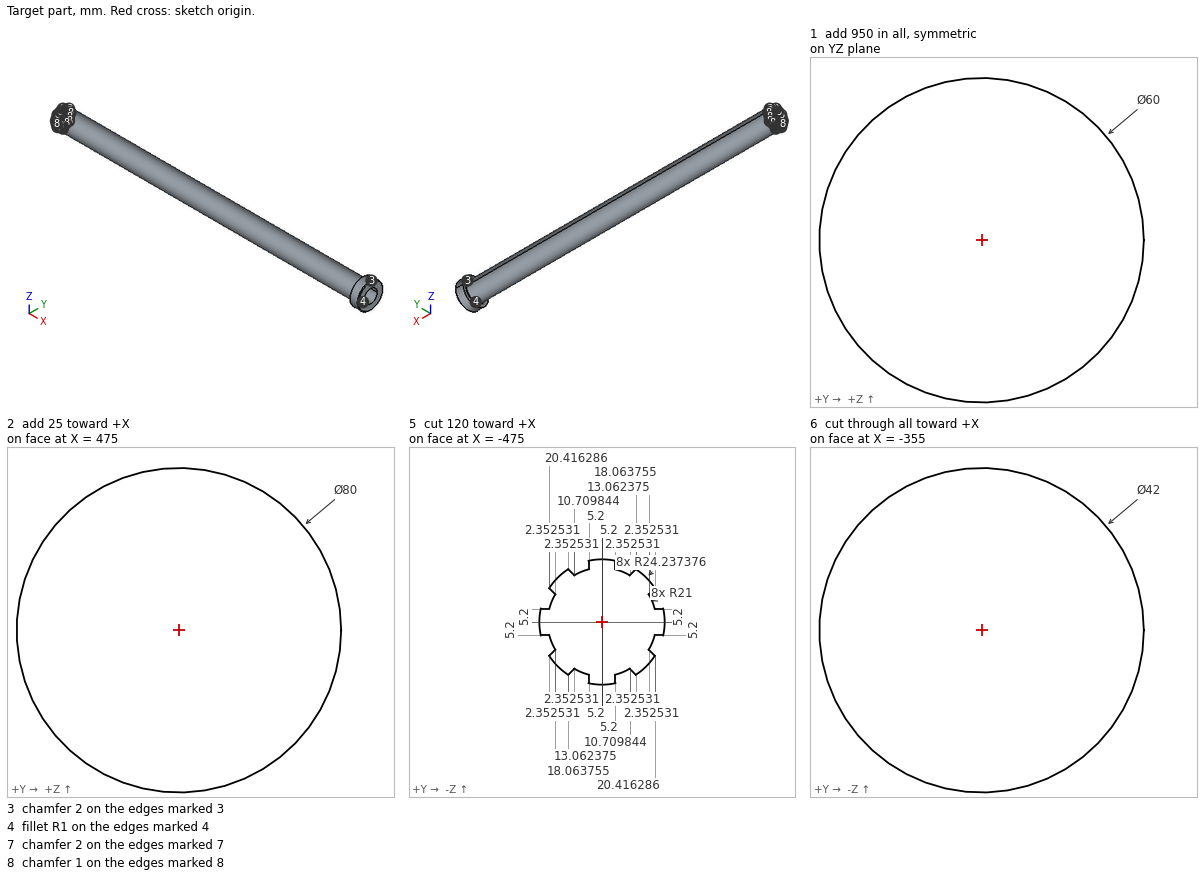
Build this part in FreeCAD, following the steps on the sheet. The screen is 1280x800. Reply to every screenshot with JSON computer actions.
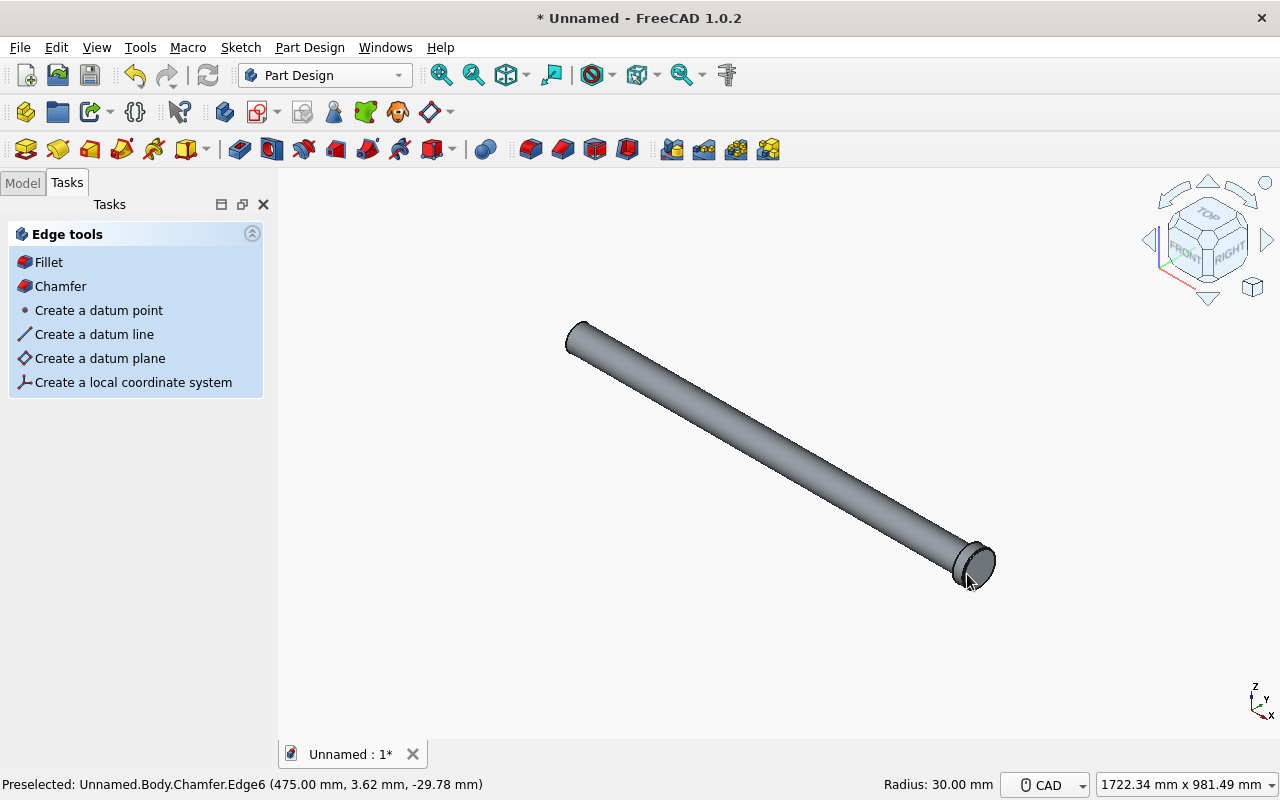
{"action": "left_click", "coordinate": [532, 150]}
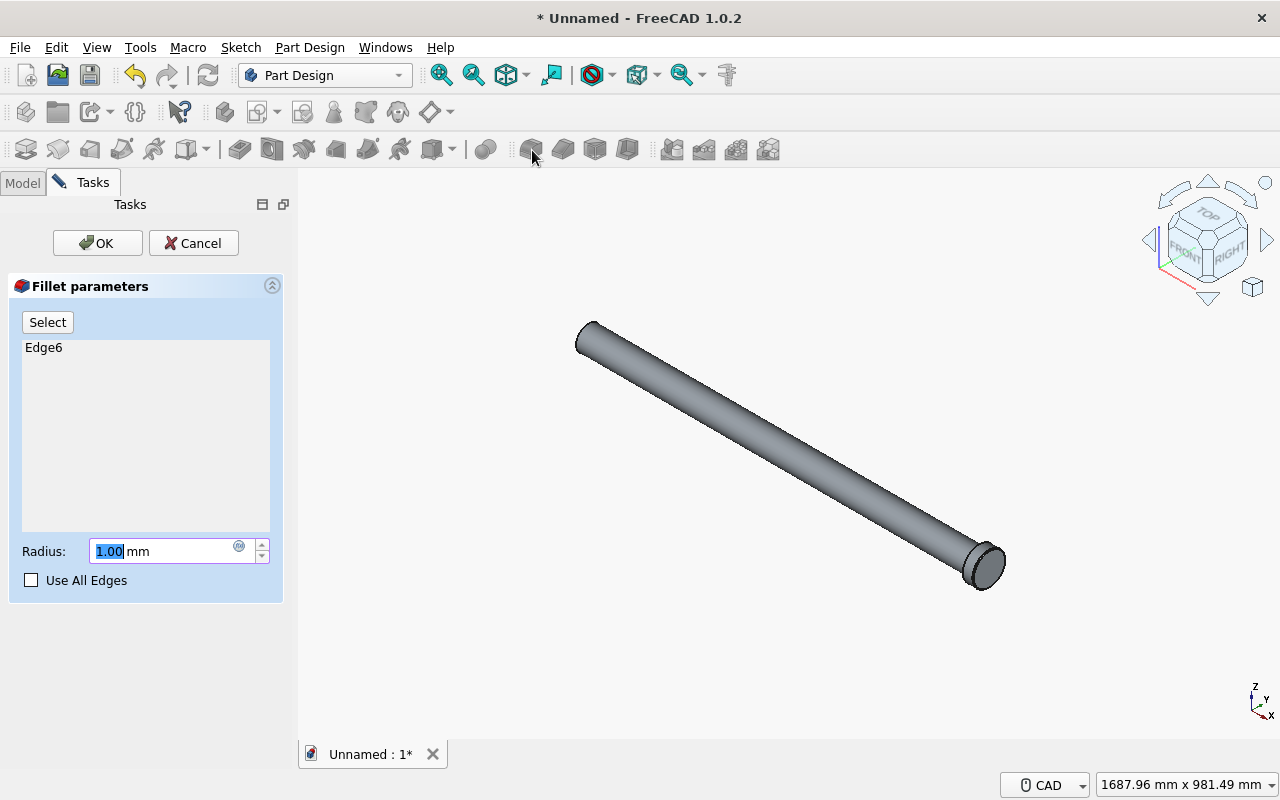
{"action": "type", "text": "1"}
{"action": "key", "text": "Tab"}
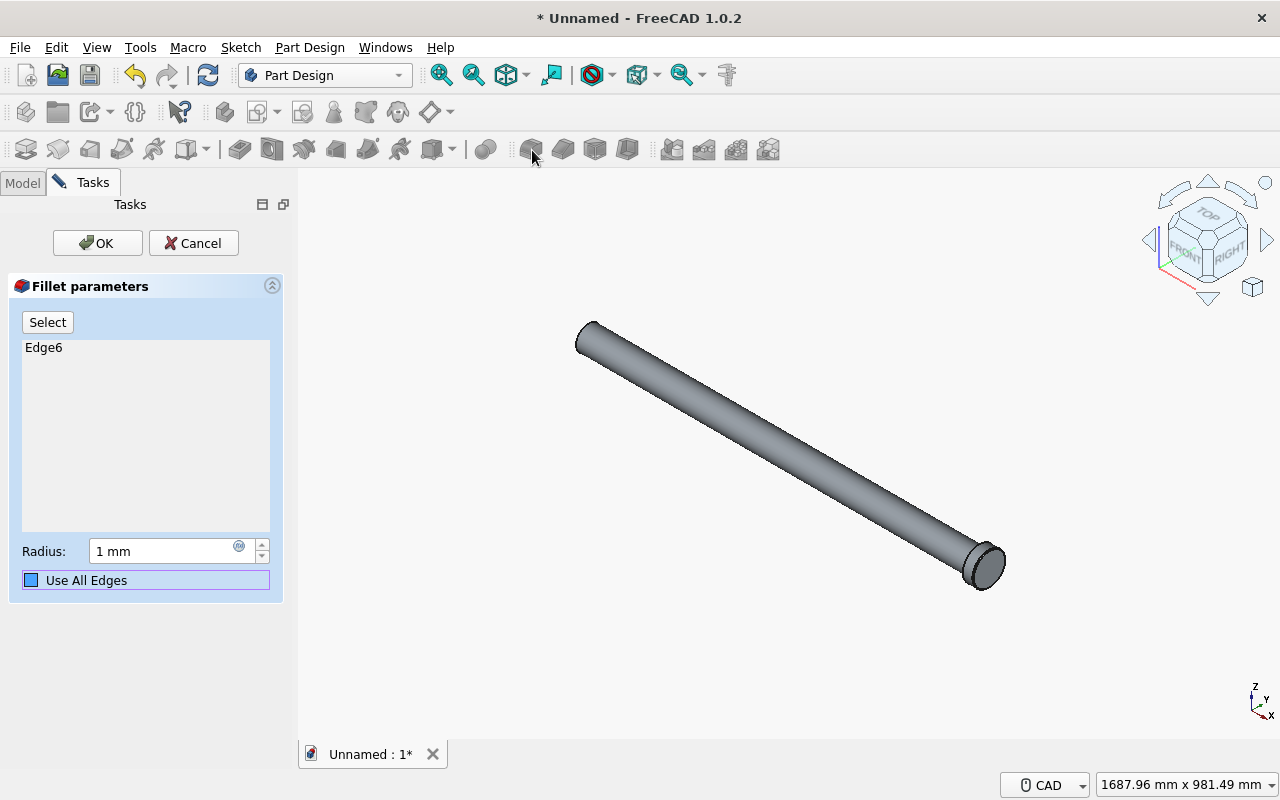
{"action": "left_click", "coordinate": [98, 243]}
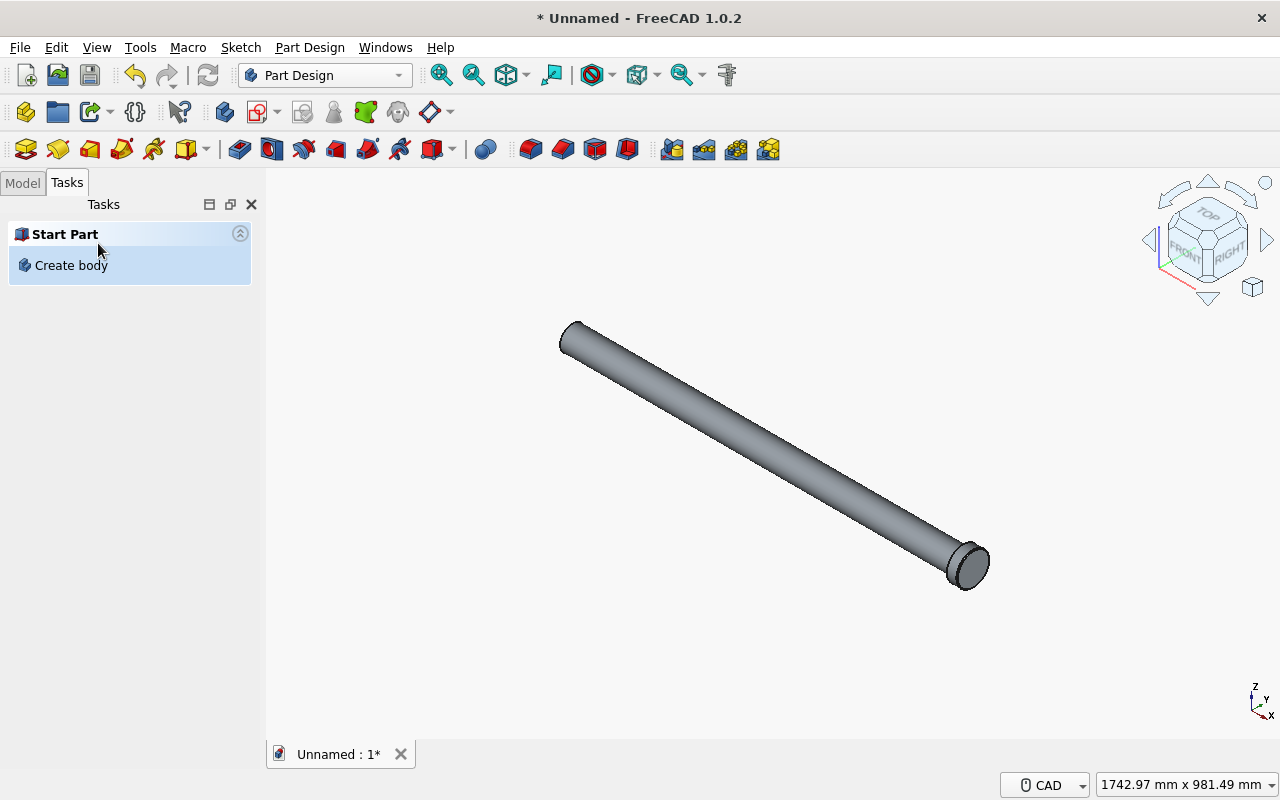
{"action": "key", "text": "6"}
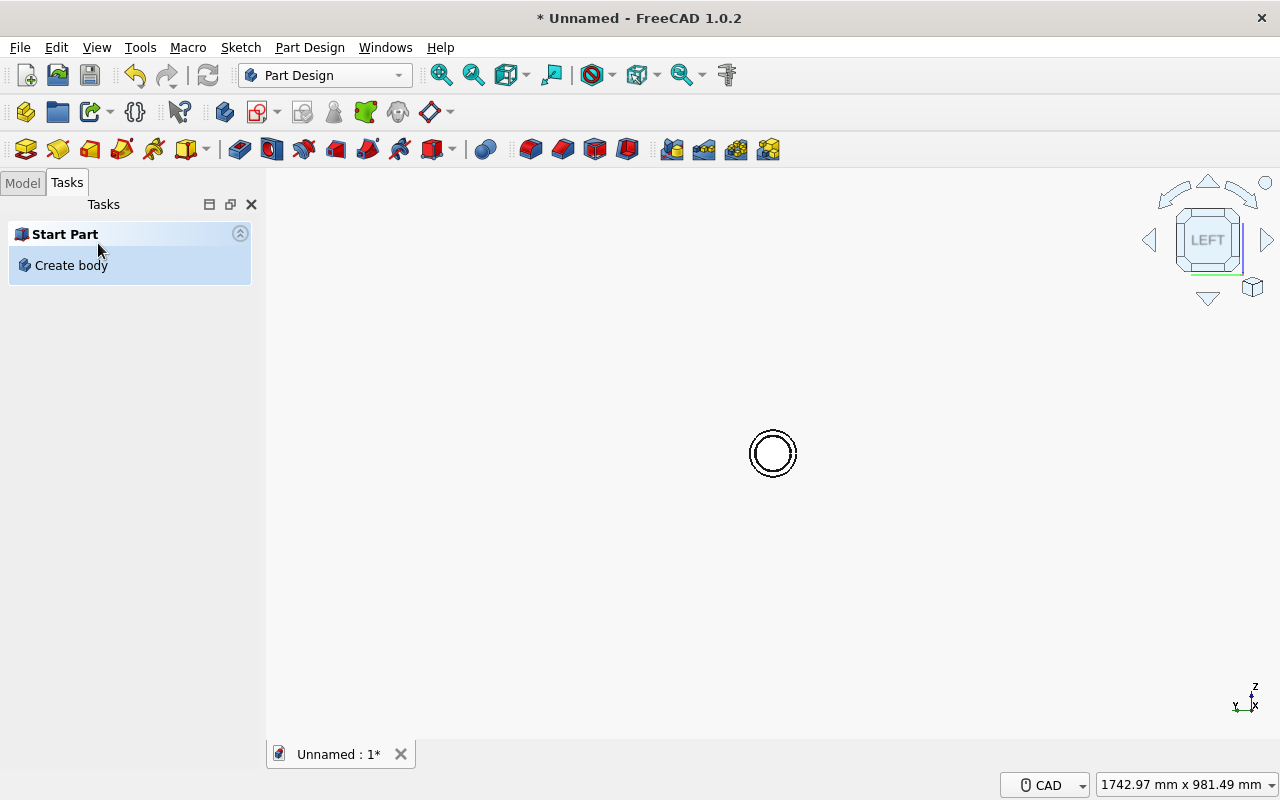
{"action": "left_click", "coordinate": [442, 76]}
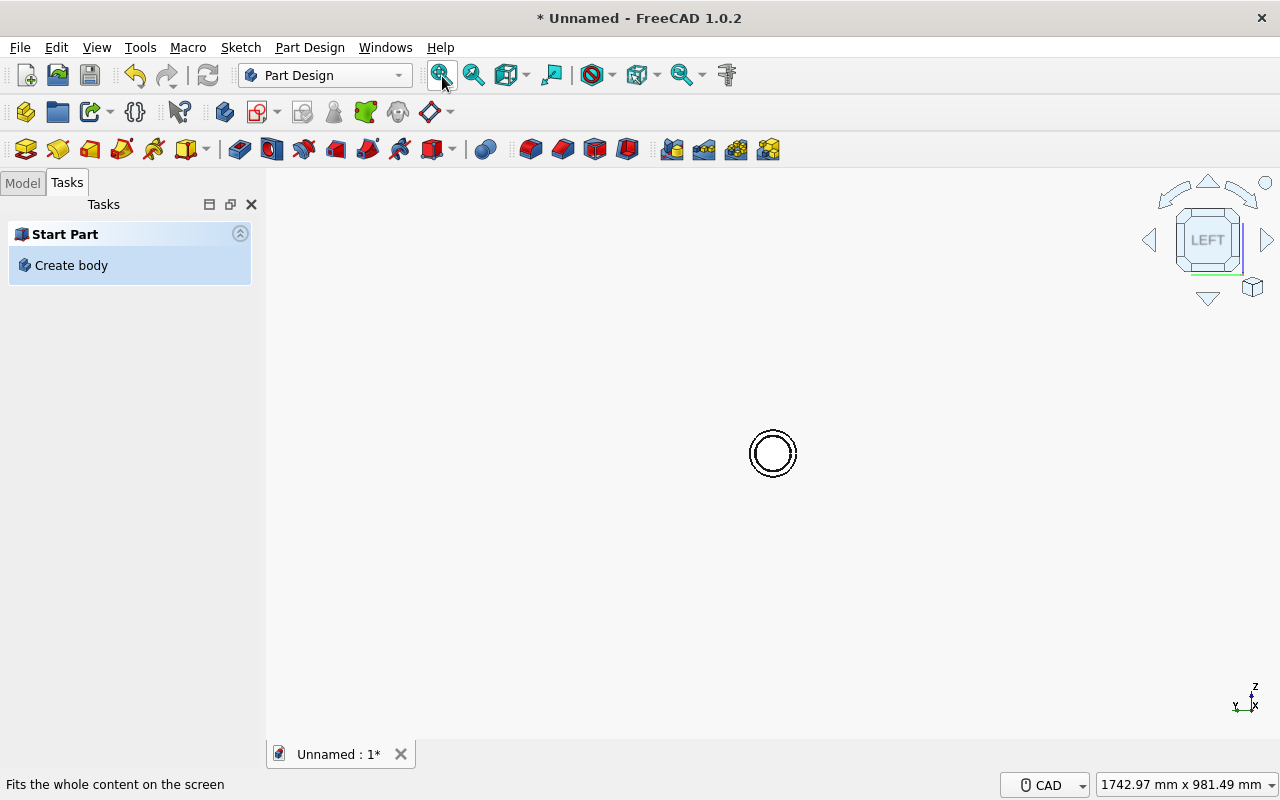
{"action": "left_click", "coordinate": [773, 452]}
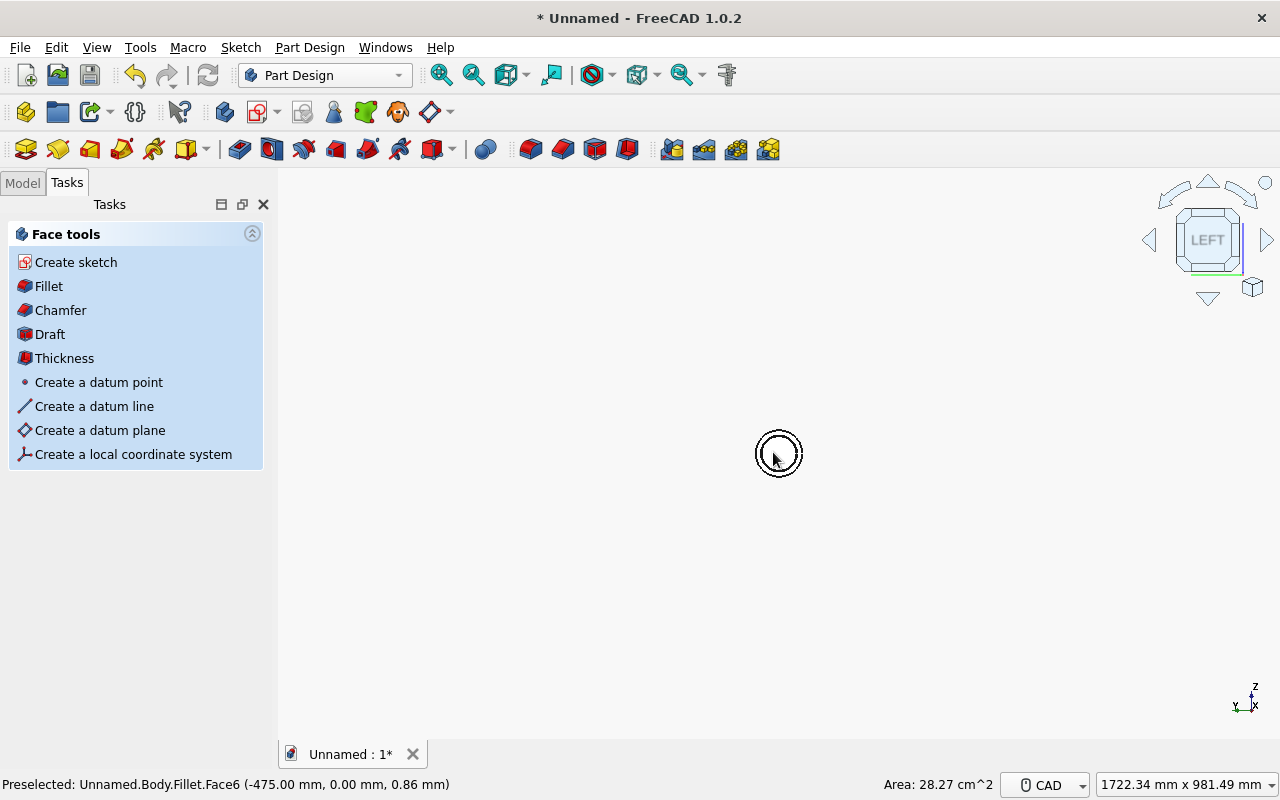
{"action": "left_click", "coordinate": [258, 112]}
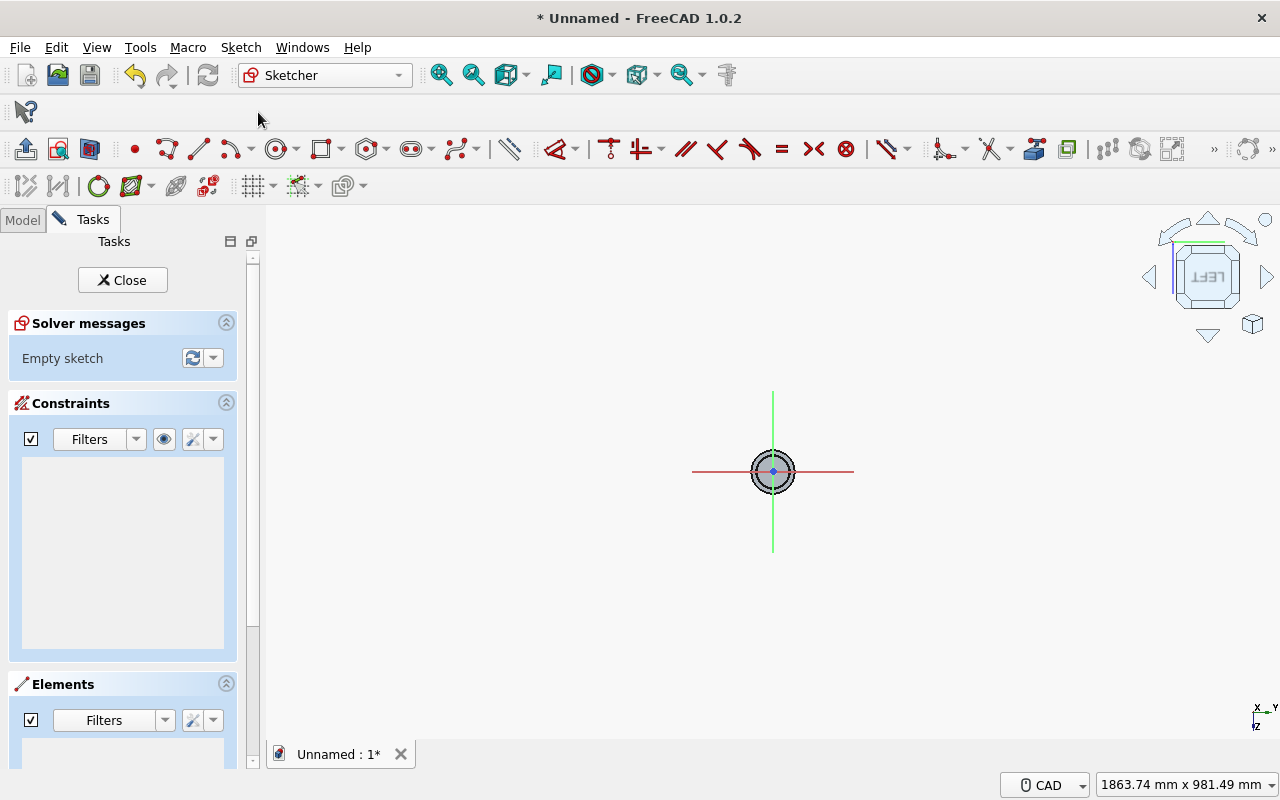
{"action": "scroll", "coordinate": [778, 472], "scroll_direction": "up", "scroll_amount": 13}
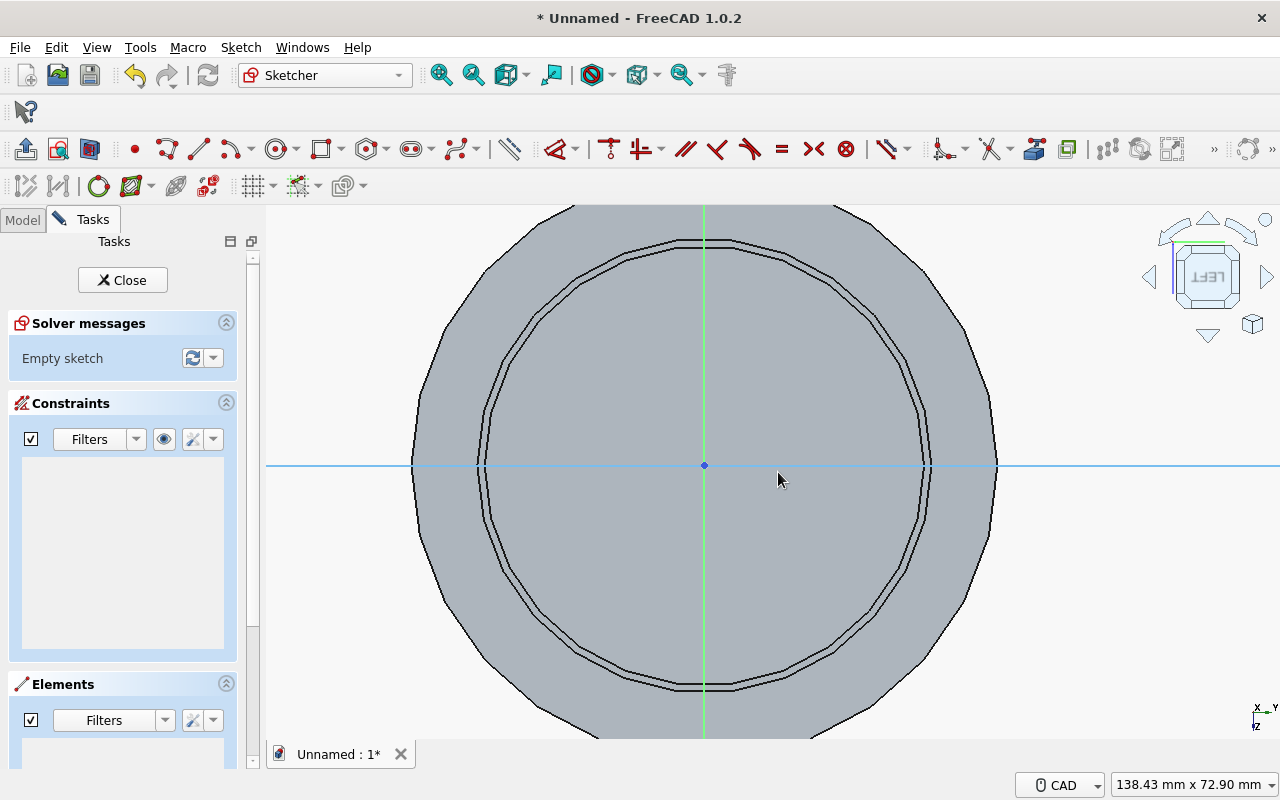
{"action": "key", "text": "g l"}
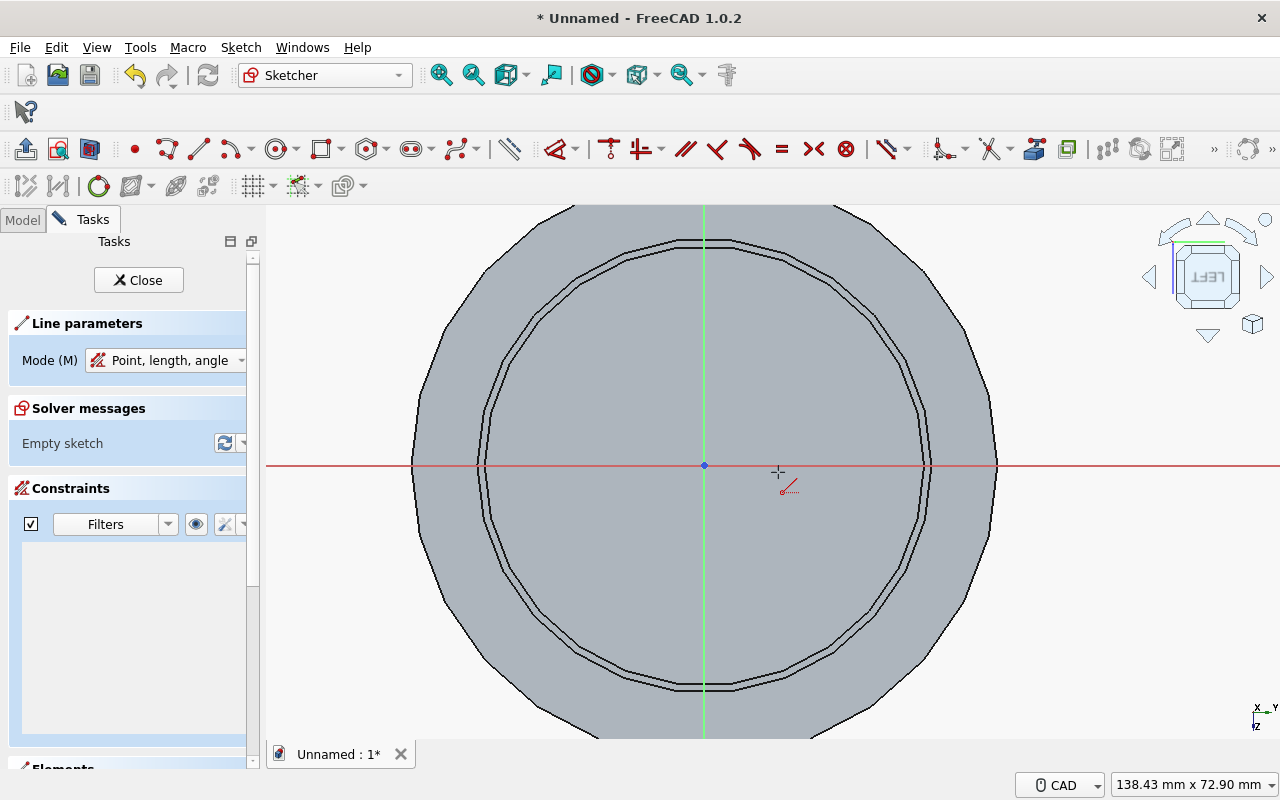
{"action": "left_click", "coordinate": [878, 428]}
{"action": "left_click", "coordinate": [853, 428]}